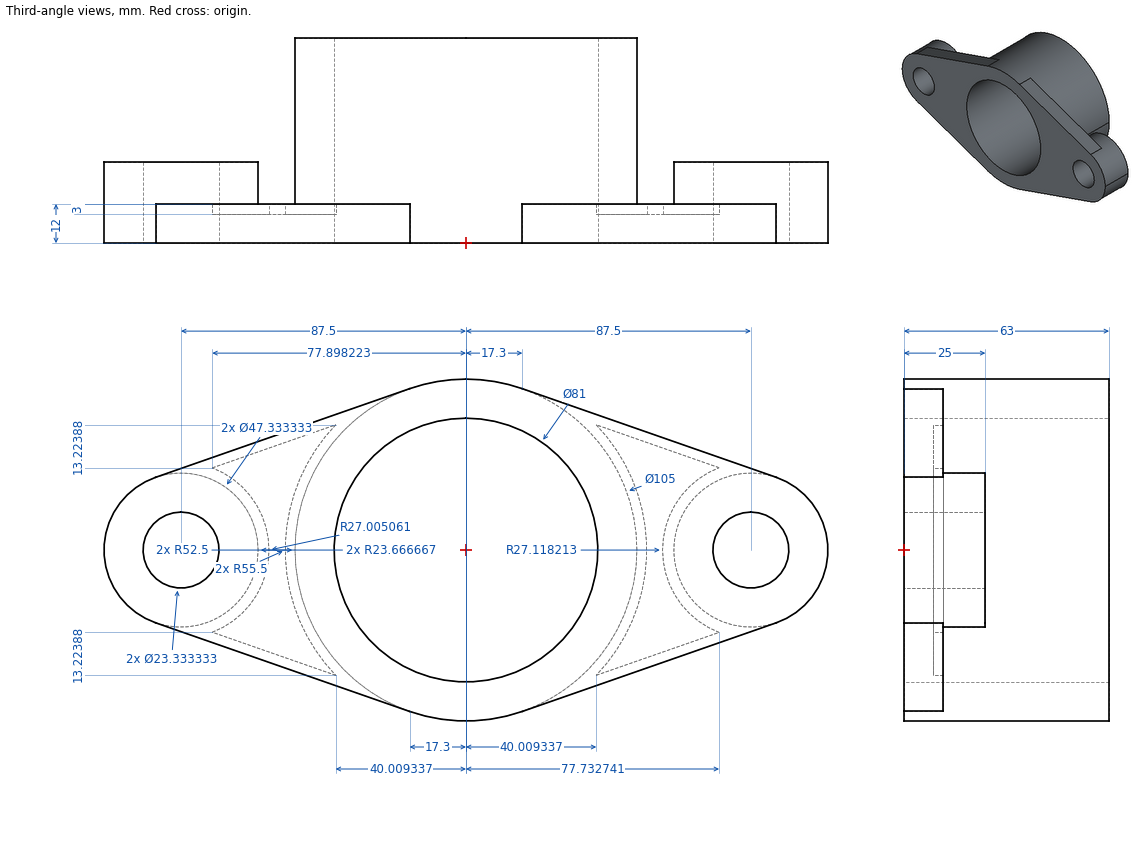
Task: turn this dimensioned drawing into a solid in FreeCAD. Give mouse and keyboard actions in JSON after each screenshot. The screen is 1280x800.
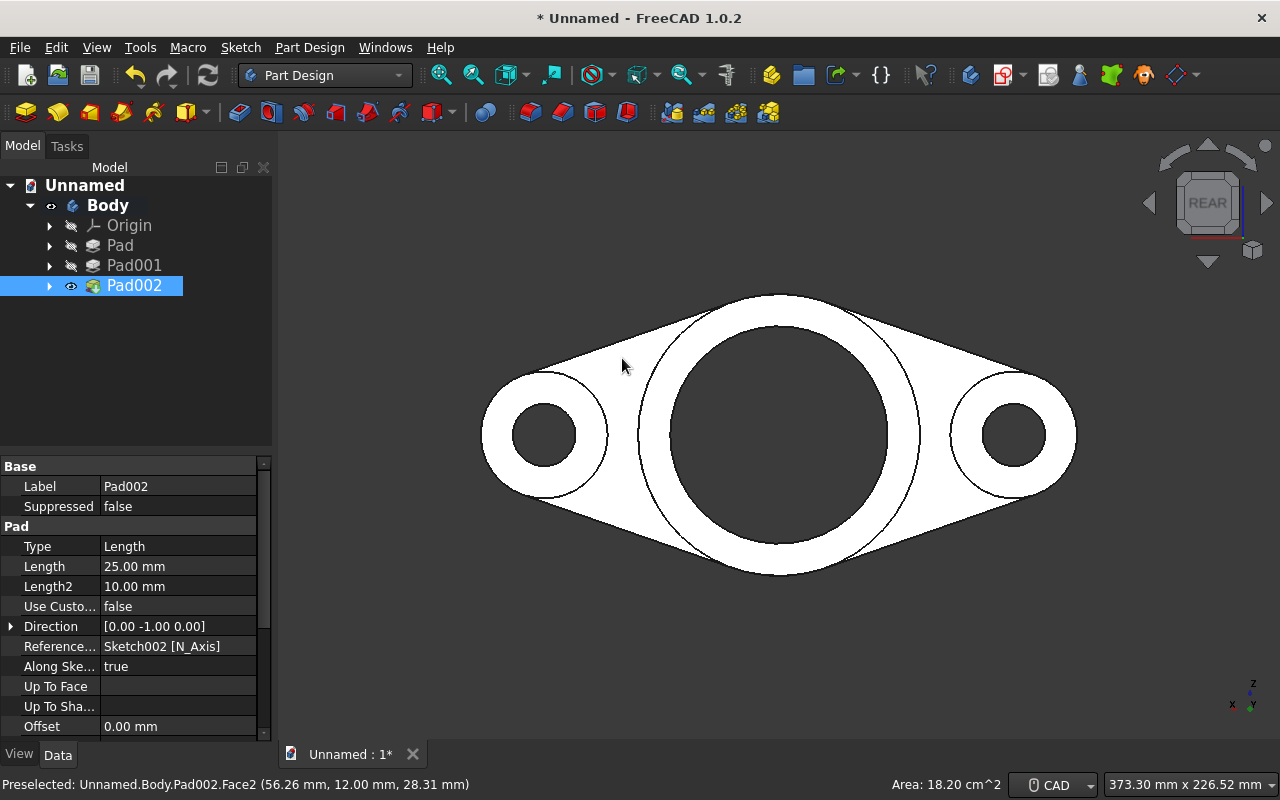
{"action": "left_click", "coordinate": [1004, 76]}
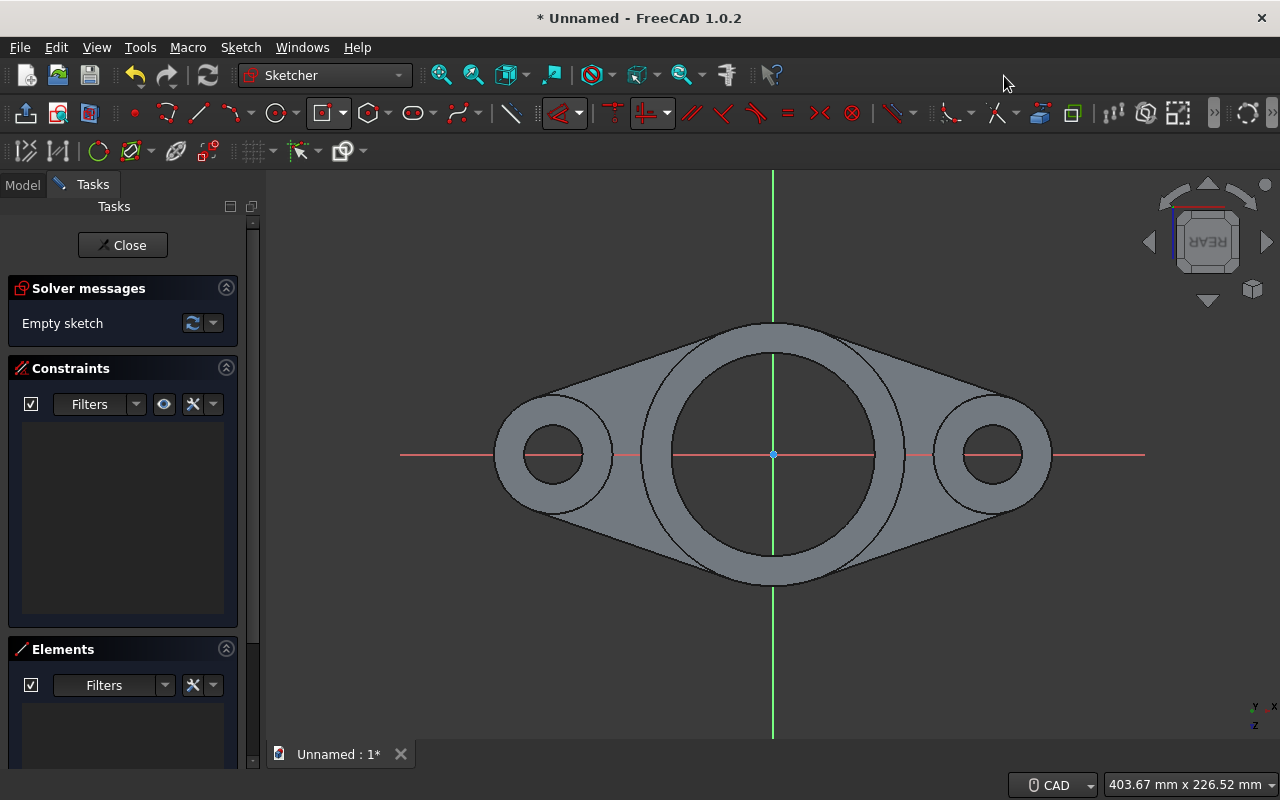
{"action": "scroll", "coordinate": [912, 454], "scroll_direction": "up", "scroll_amount": 2}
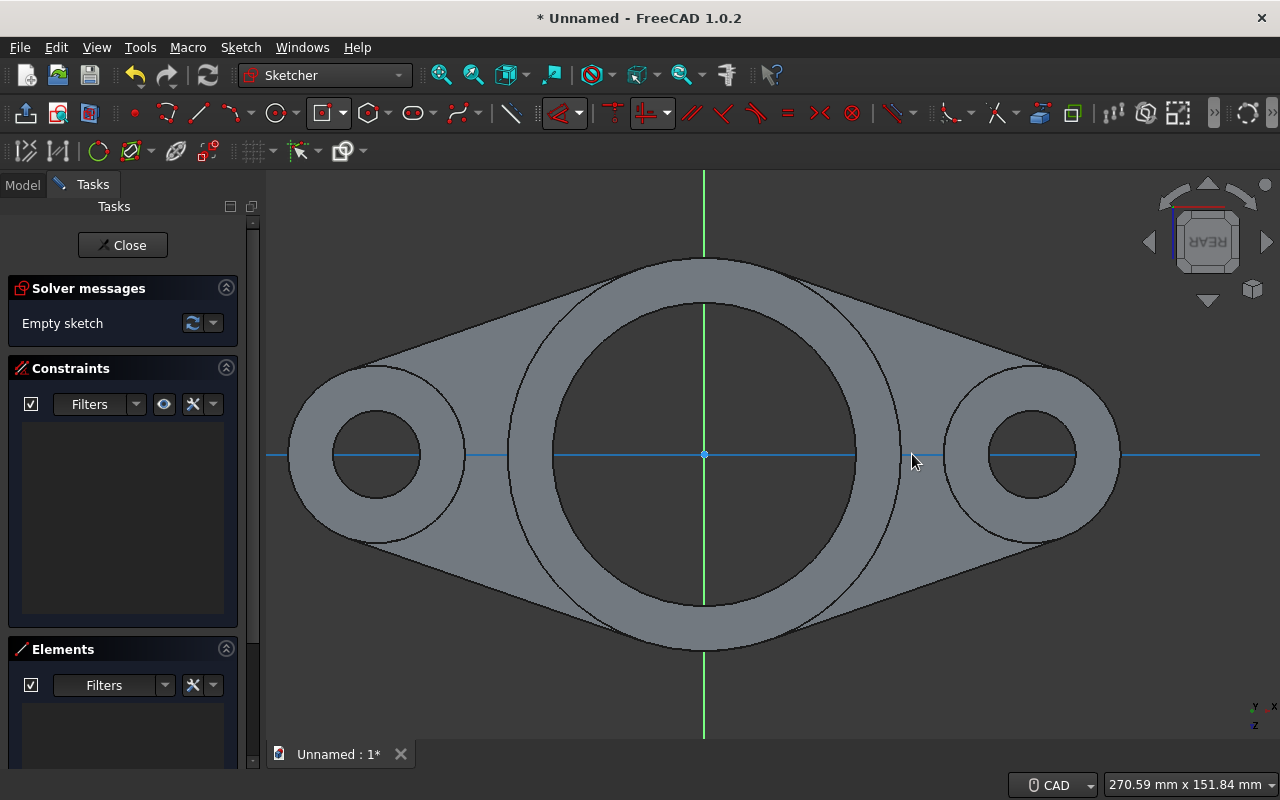
{"action": "key", "text": "g l"}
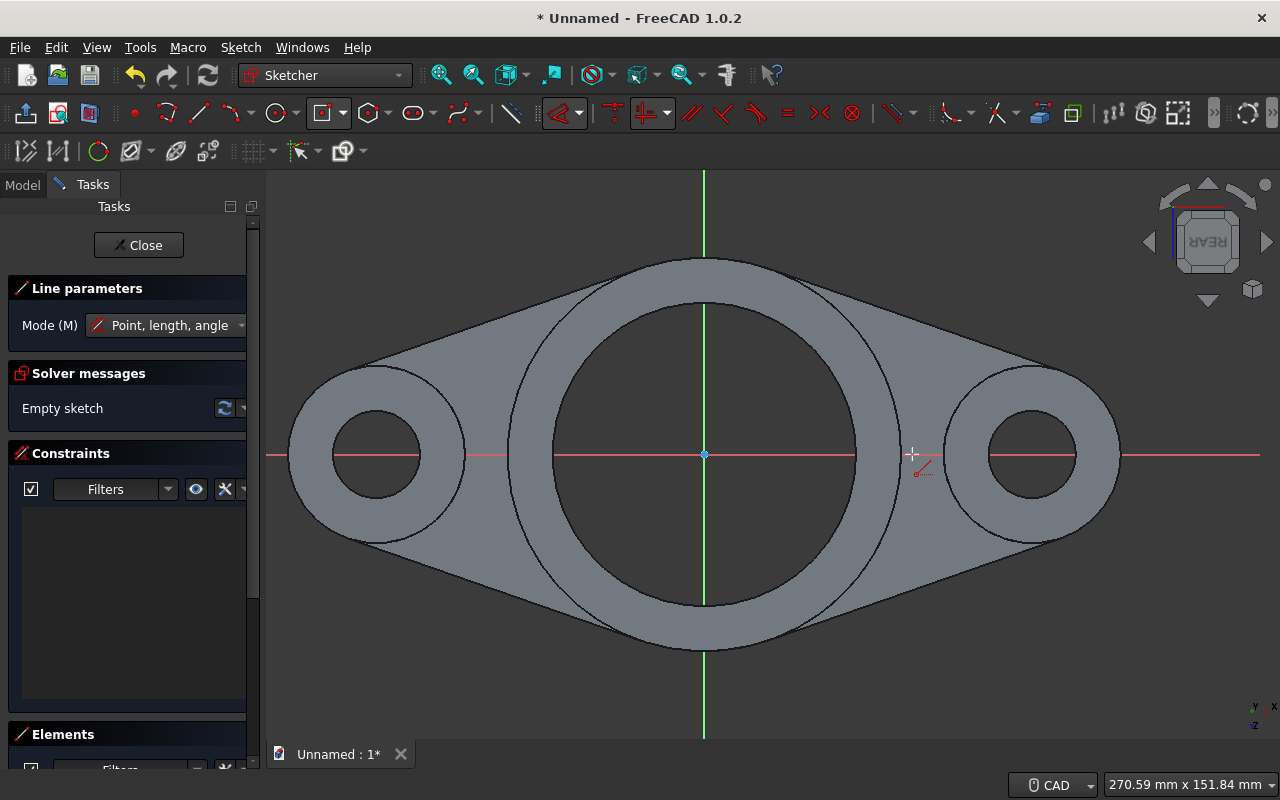
{"action": "left_click", "coordinate": [554, 310]}
{"action": "left_click", "coordinate": [412, 360]}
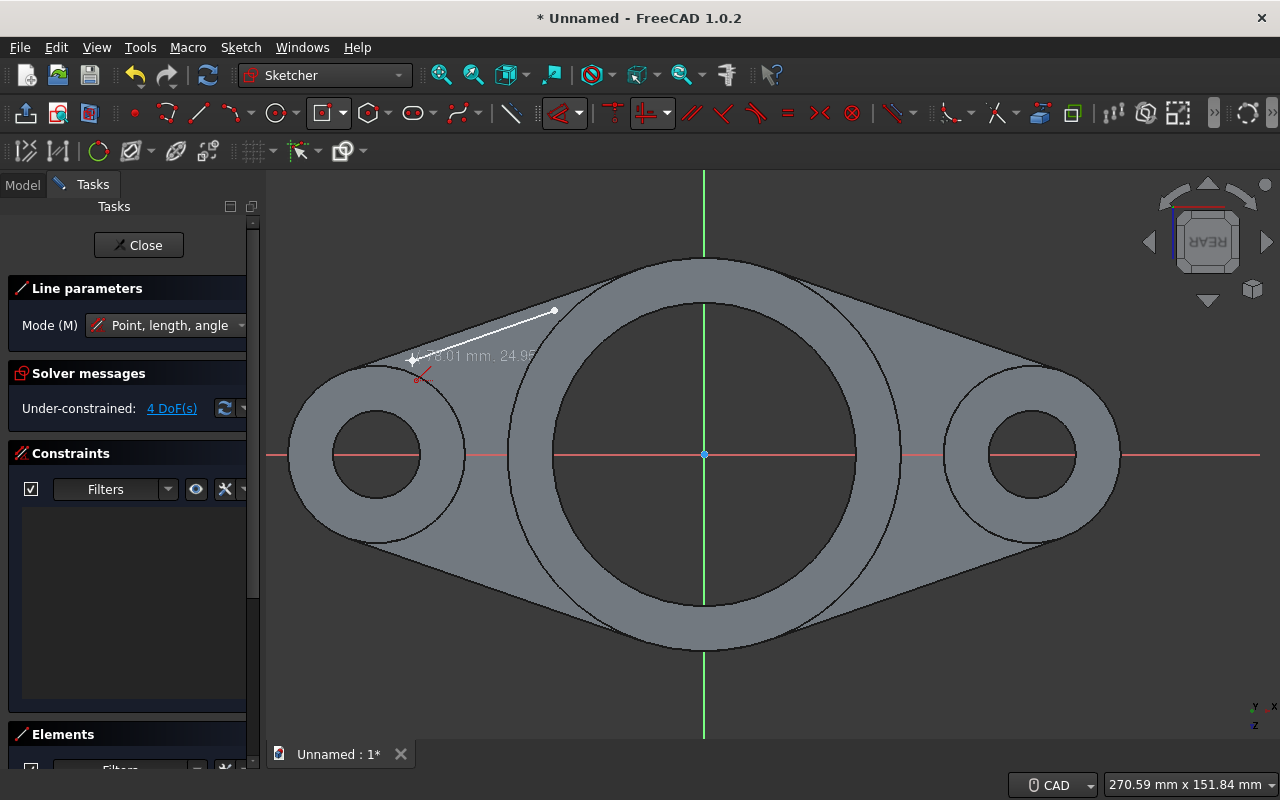
{"action": "left_click", "coordinate": [412, 549]}
{"action": "left_click", "coordinate": [554, 599]}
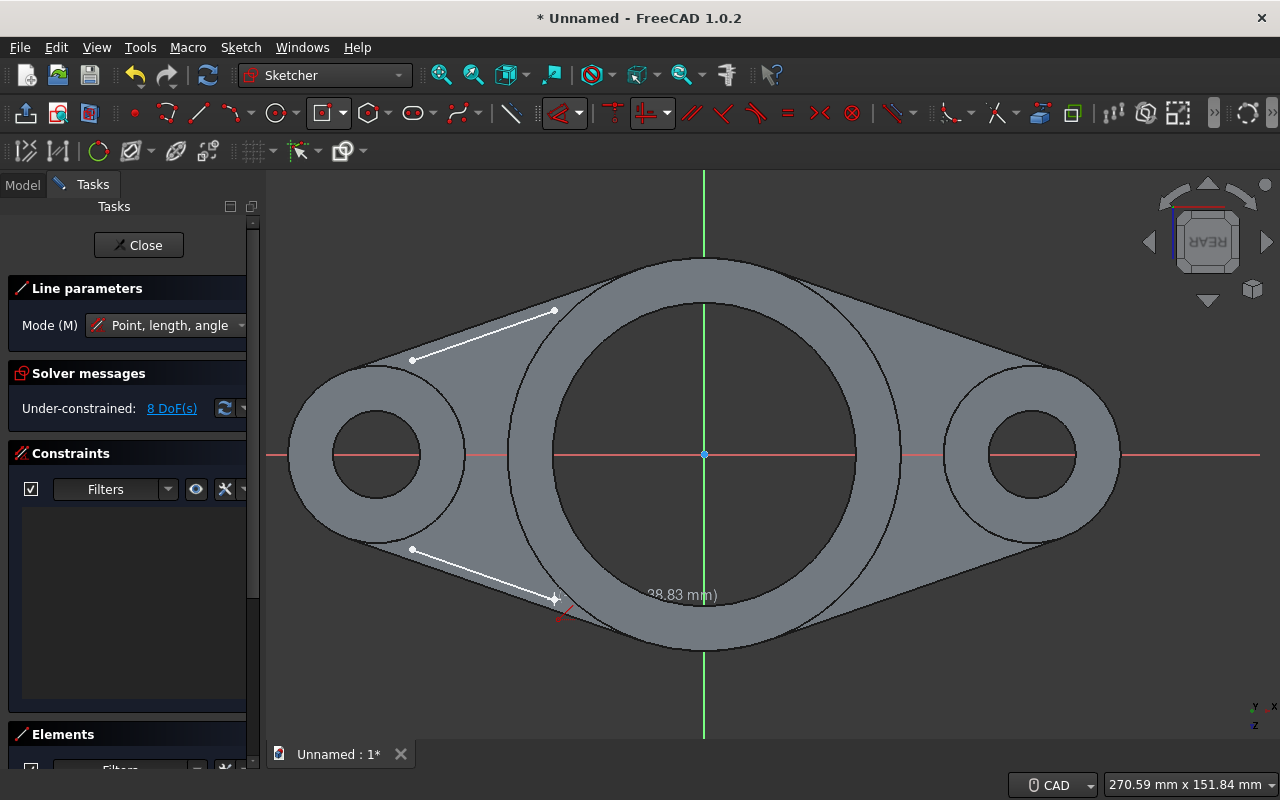
{"action": "left_click", "coordinate": [232, 114]}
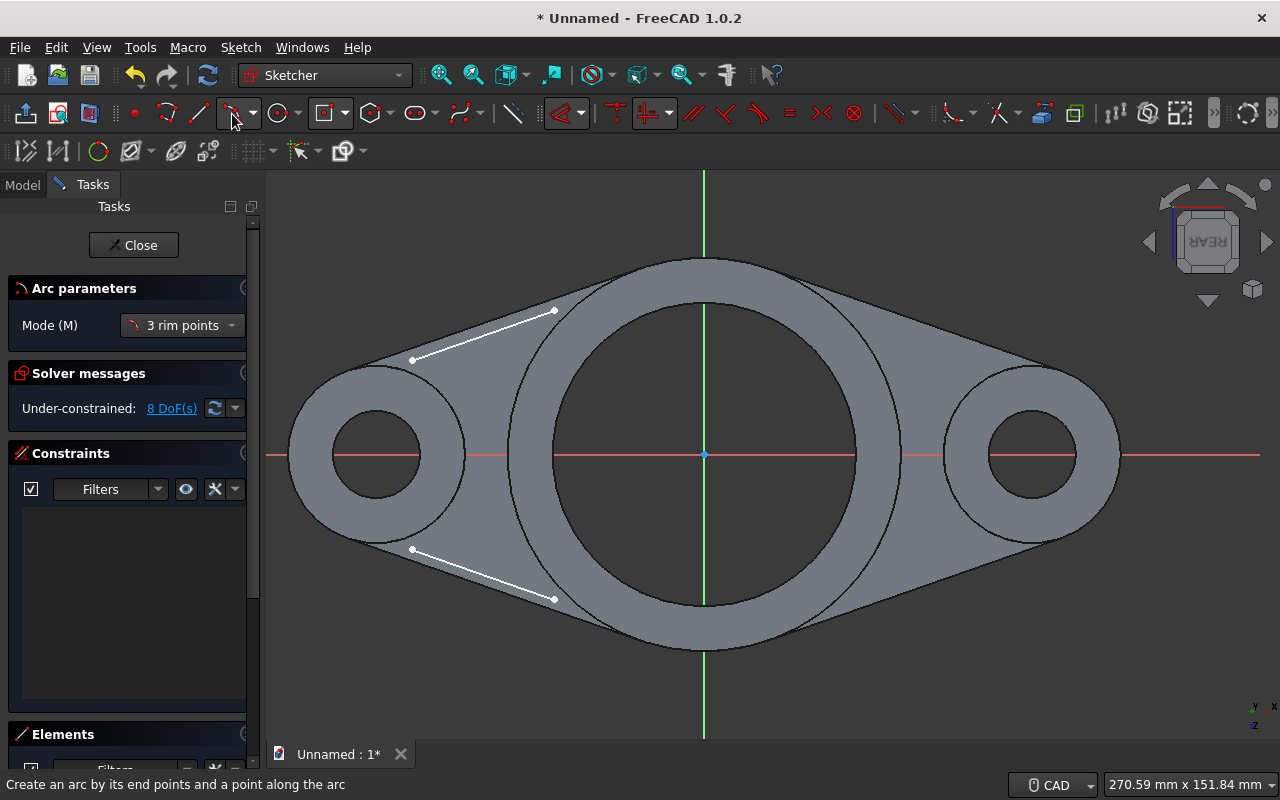
{"action": "left_click", "coordinate": [412, 361]}
{"action": "left_click", "coordinate": [412, 550]}
{"action": "left_click", "coordinate": [475, 479]}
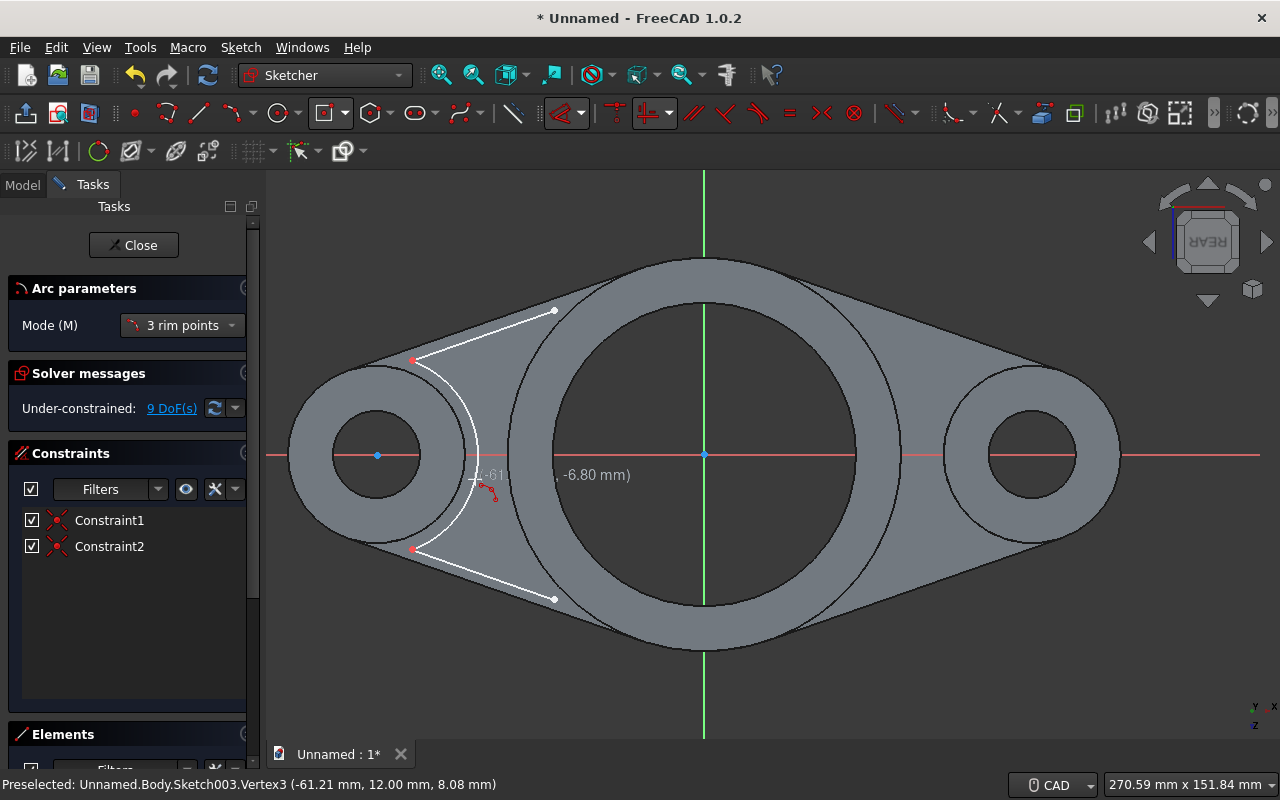
{"action": "left_click", "coordinate": [554, 600]}
{"action": "left_click", "coordinate": [554, 311]}
{"action": "left_click", "coordinate": [499, 423]}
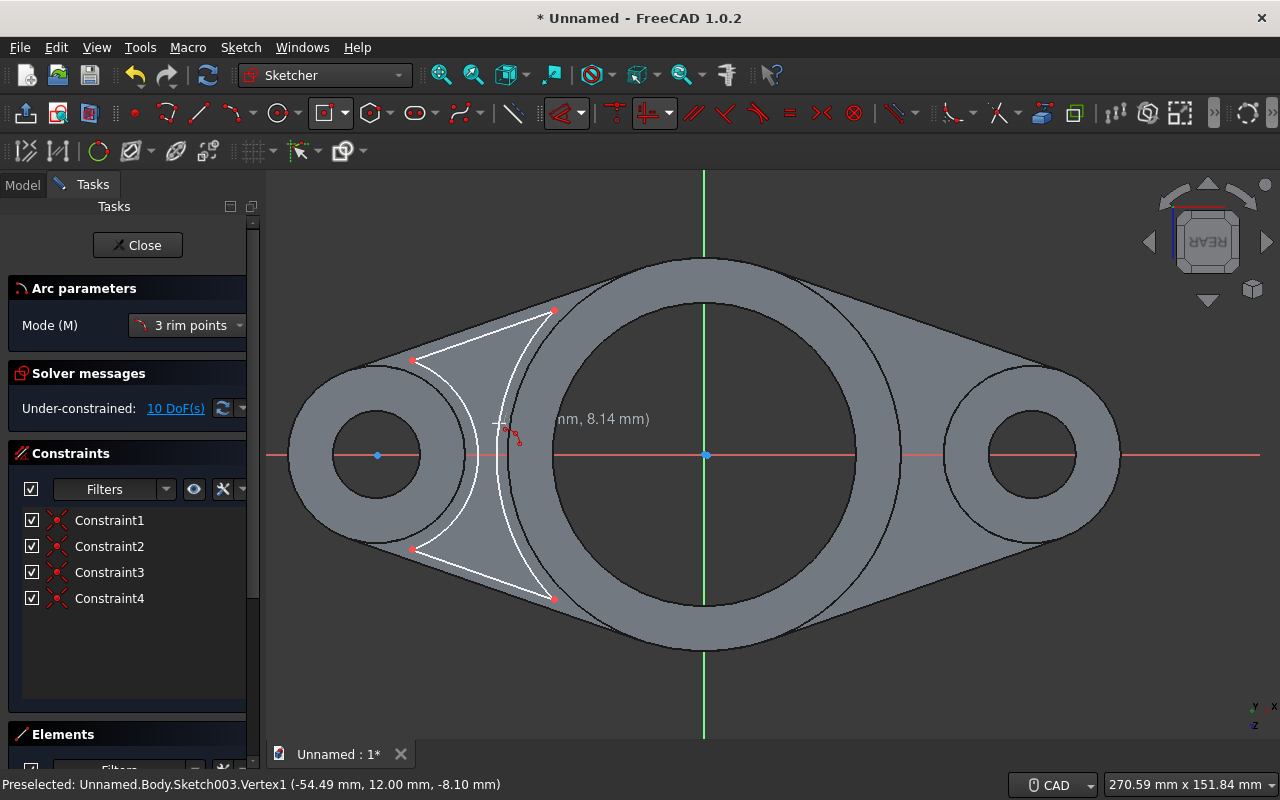
{"action": "key", "text": "g l"}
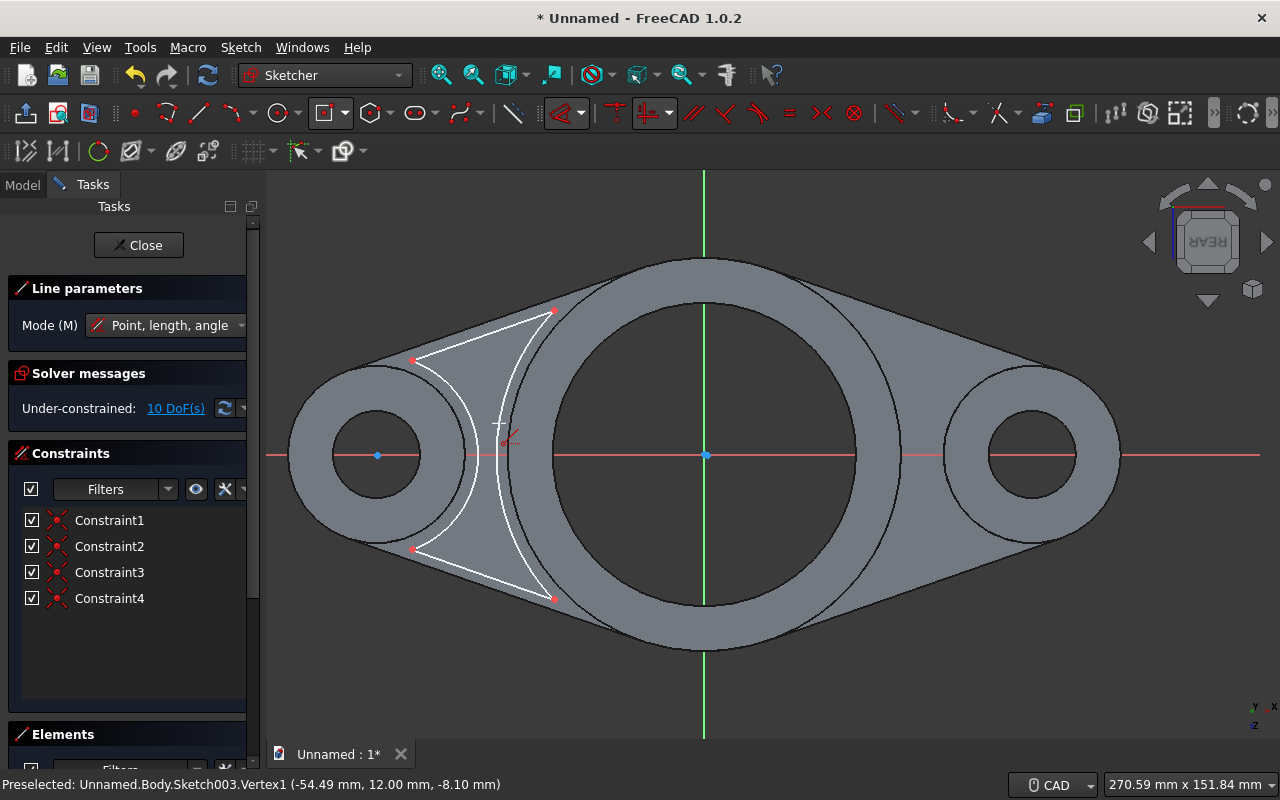
{"action": "left_click", "coordinate": [996, 360]}
{"action": "left_click", "coordinate": [854, 310]}